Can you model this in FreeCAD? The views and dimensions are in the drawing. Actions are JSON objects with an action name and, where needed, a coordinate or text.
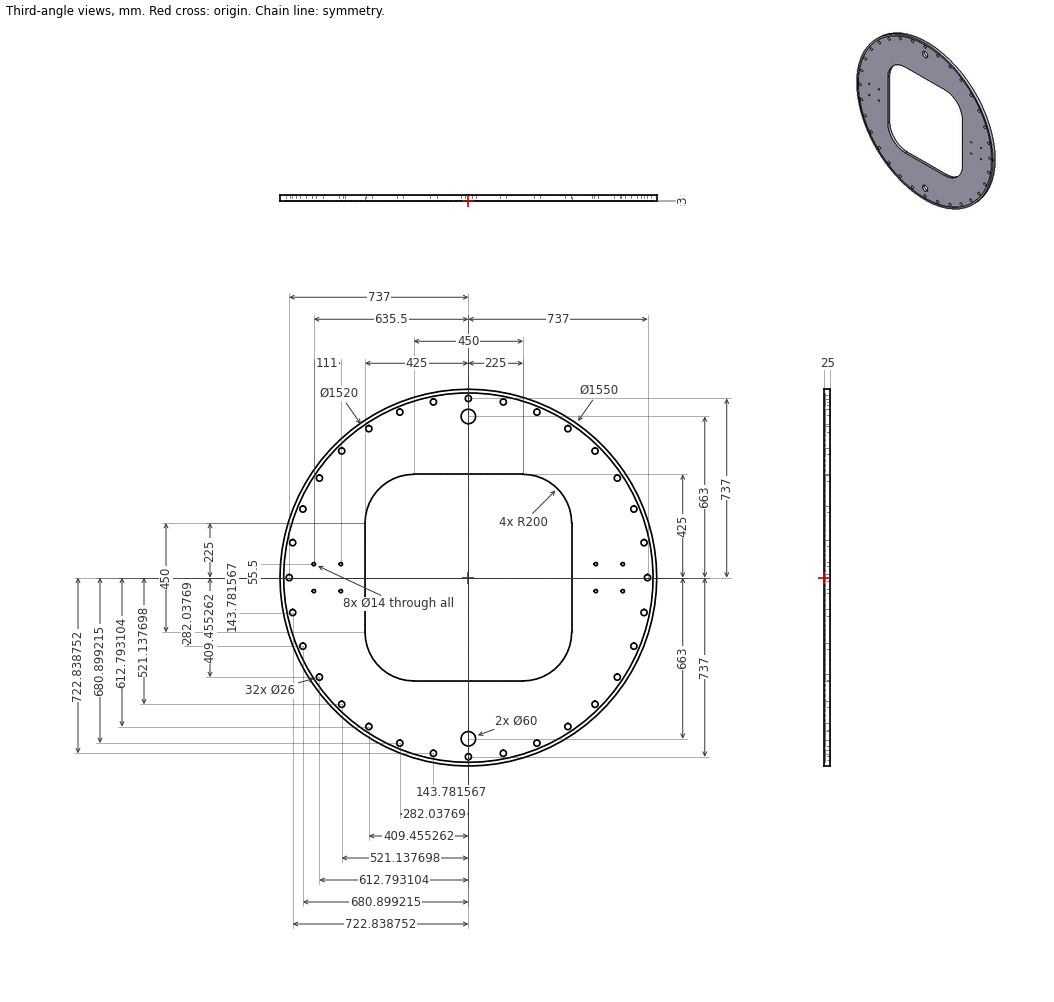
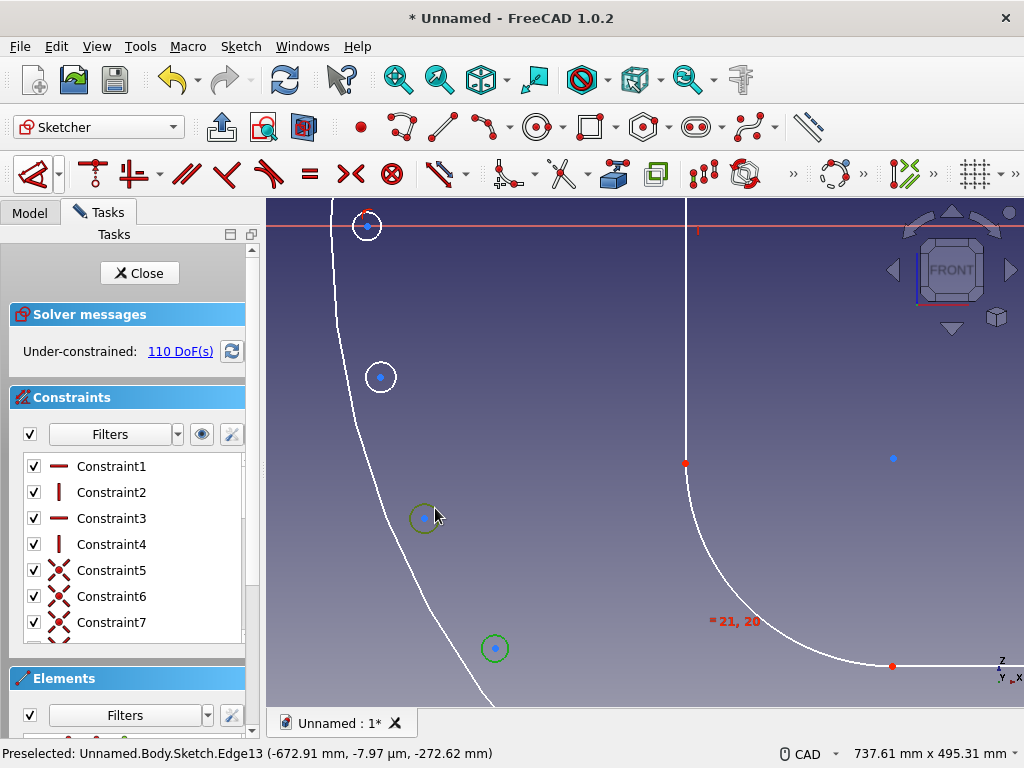
{"action": "left_click", "coordinate": [391, 367]}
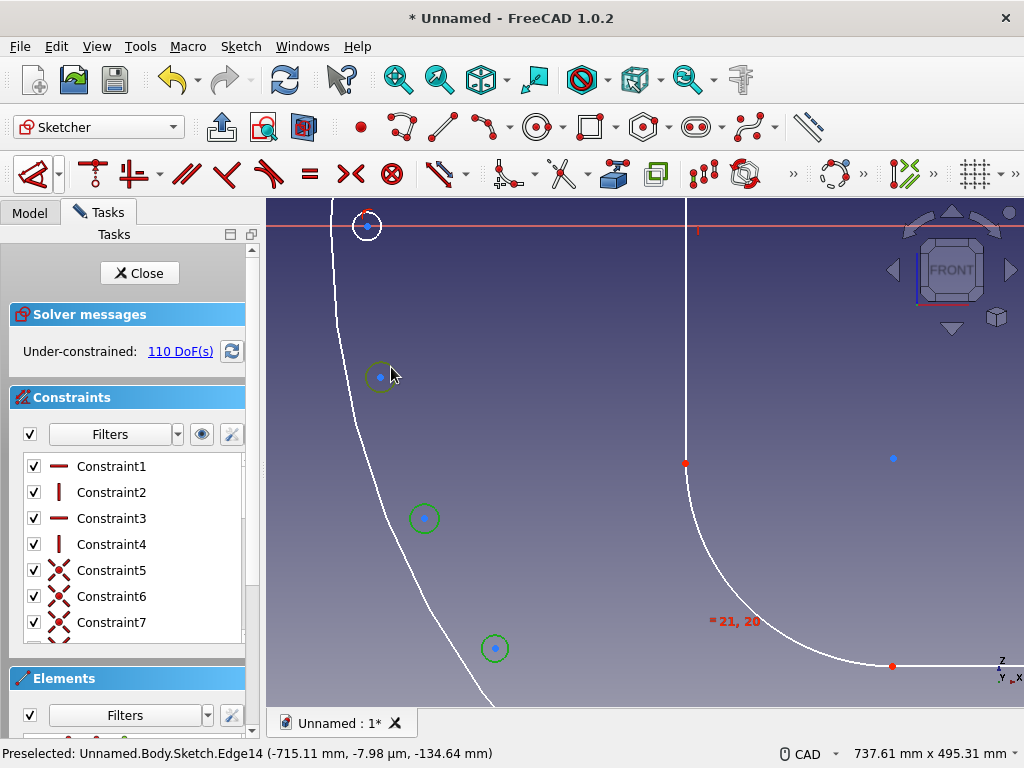
{"action": "scroll", "coordinate": [438, 510], "scroll_direction": "down", "scroll_amount": 8}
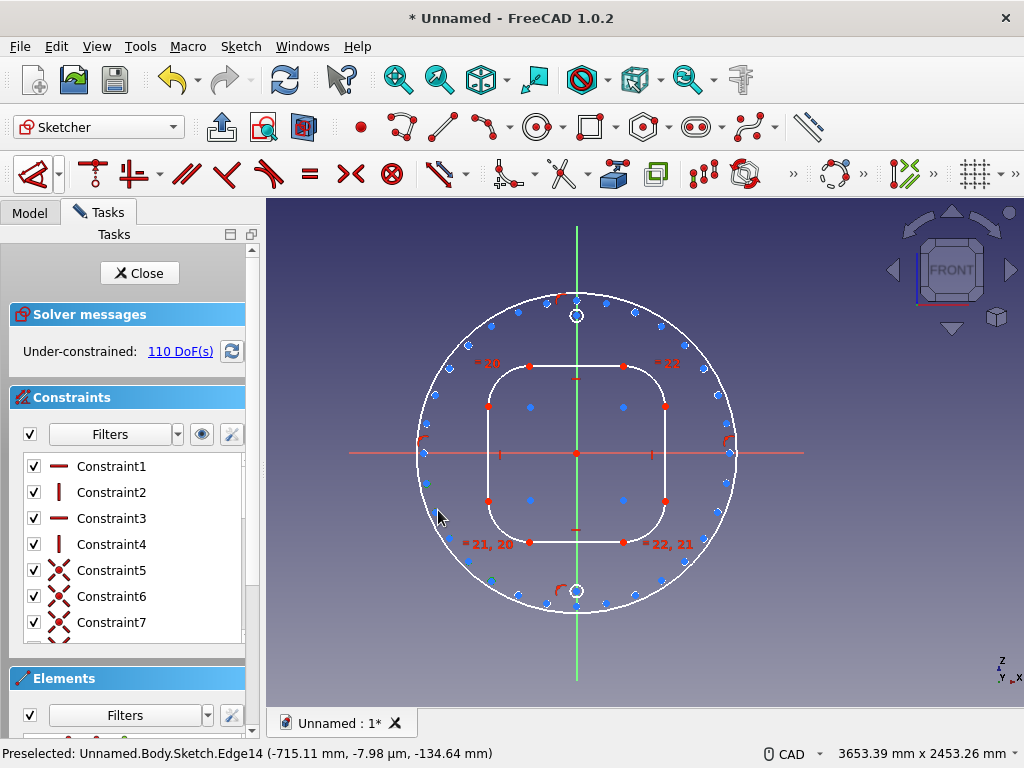
{"action": "scroll", "coordinate": [520, 593], "scroll_direction": "up", "scroll_amount": 8}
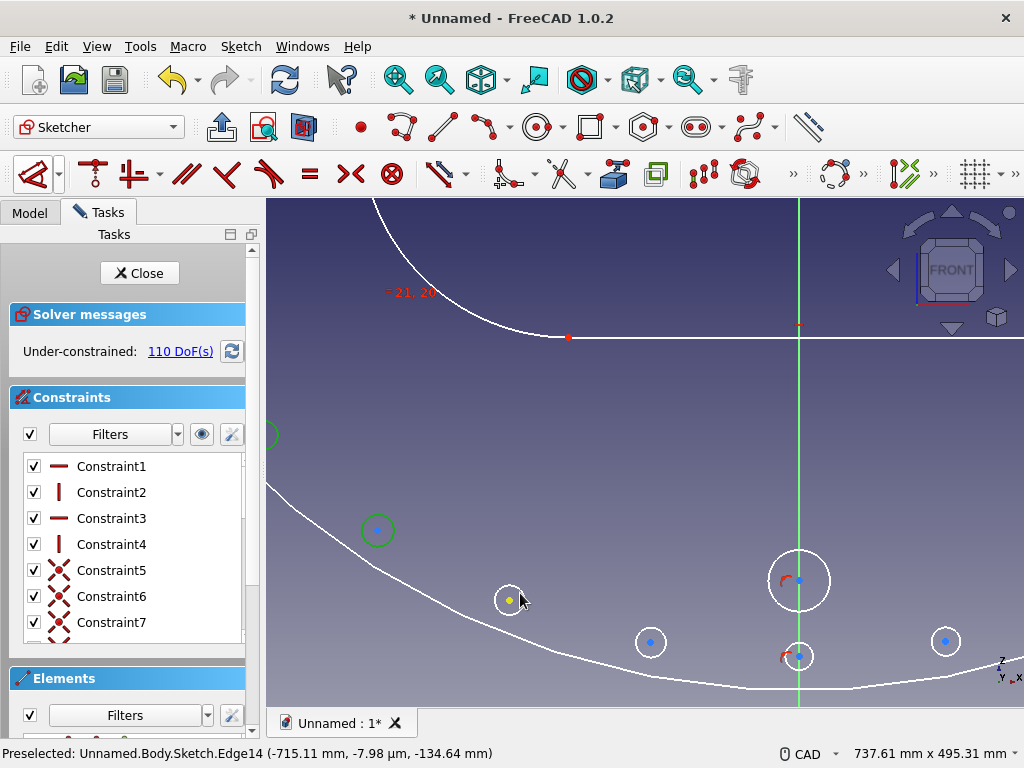
{"action": "left_click", "coordinate": [520, 590]}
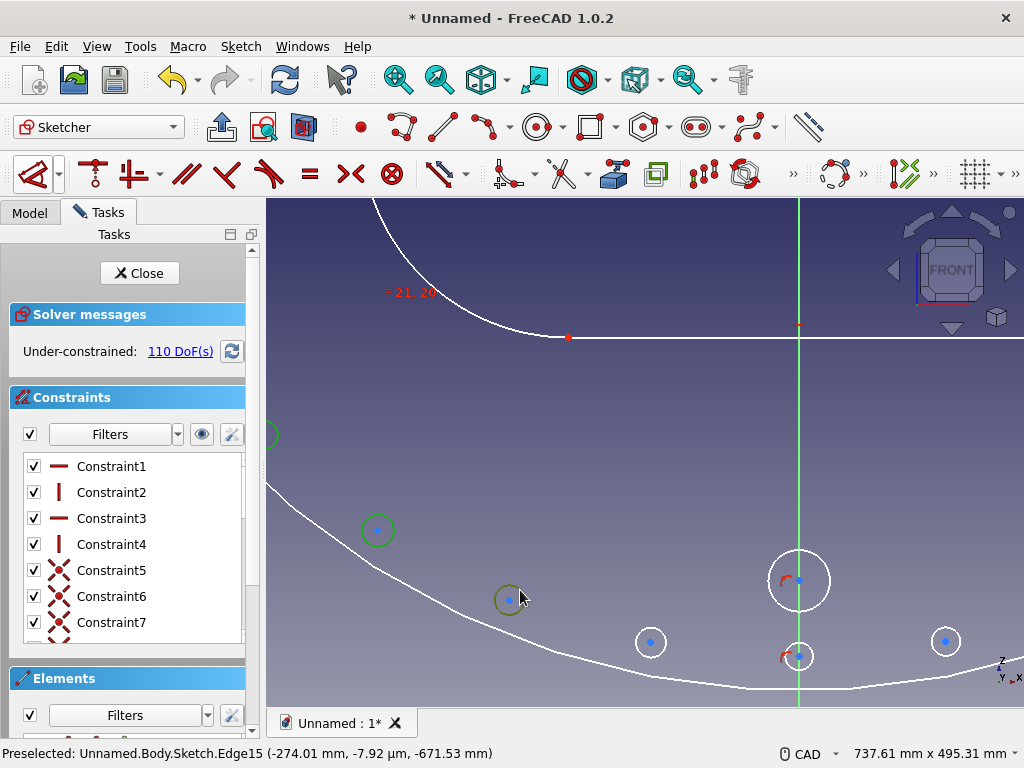
{"action": "left_click", "coordinate": [662, 632]}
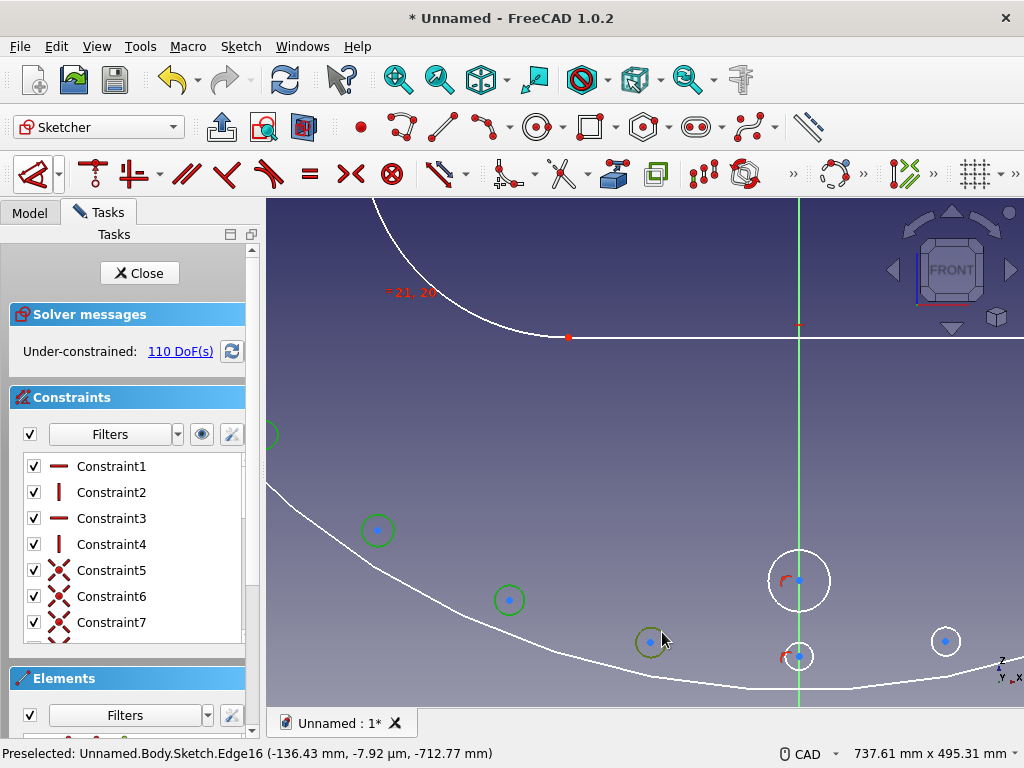
{"action": "scroll", "coordinate": [809, 647], "scroll_direction": "up", "scroll_amount": 2}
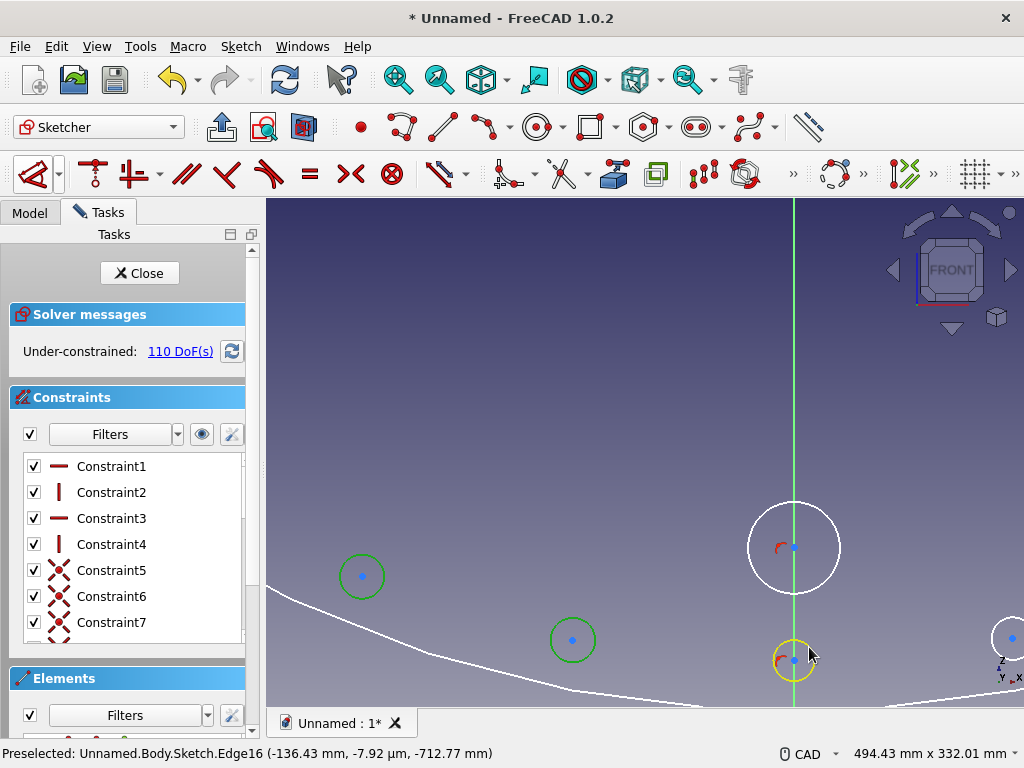
{"action": "left_click", "coordinate": [808, 646]}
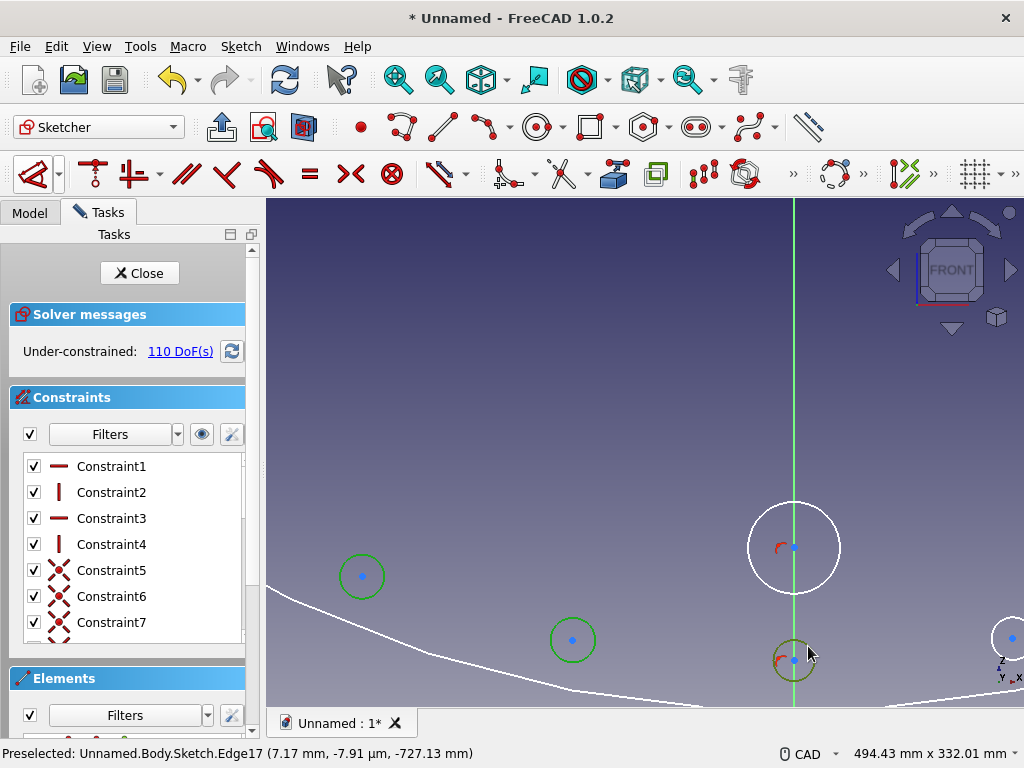
{"action": "scroll", "coordinate": [542, 597], "scroll_direction": "down", "scroll_amount": 10}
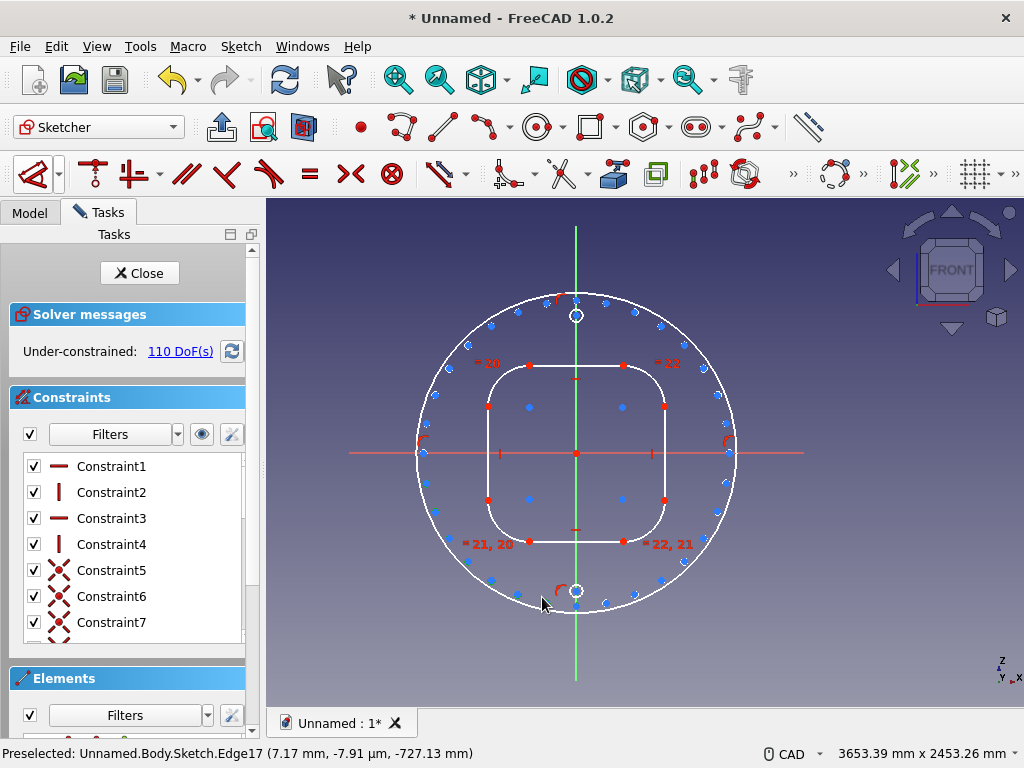
{"action": "scroll", "coordinate": [426, 451], "scroll_direction": "up", "scroll_amount": 10}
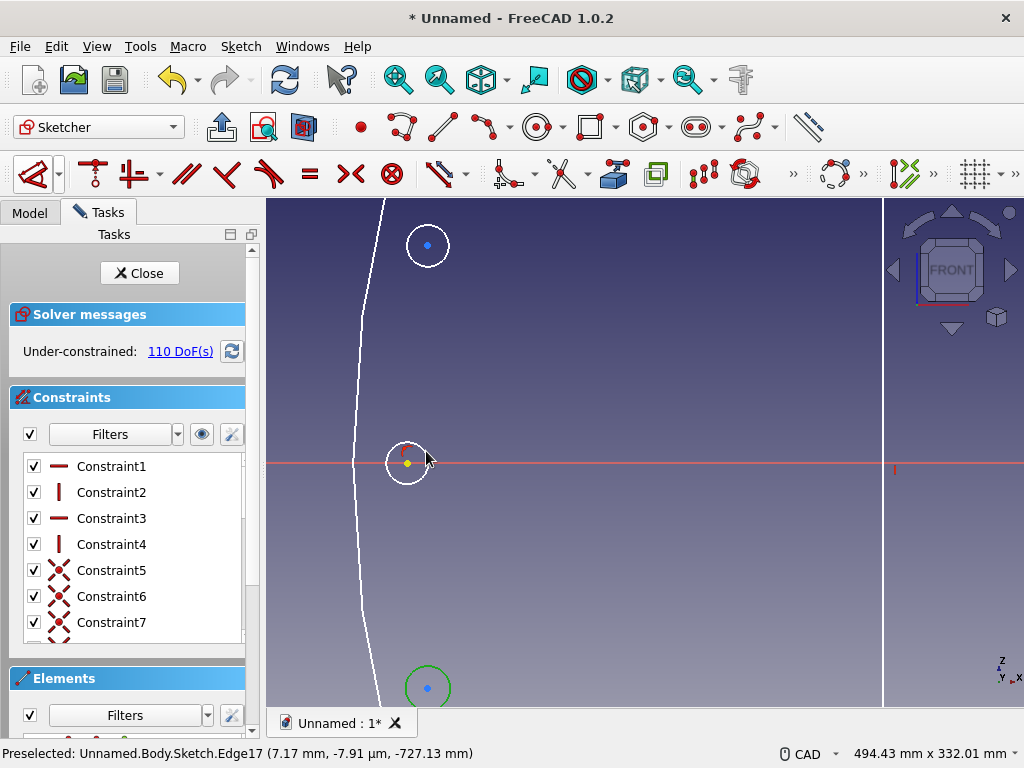
{"action": "left_click", "coordinate": [422, 448]}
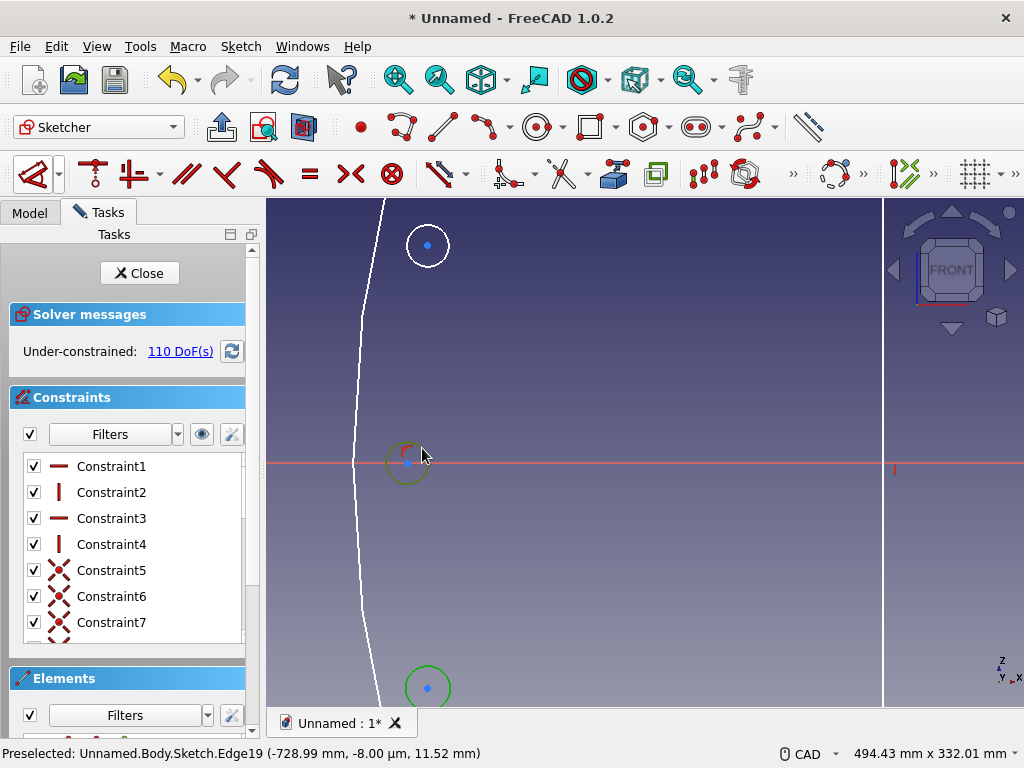
{"action": "left_click", "coordinate": [443, 231]}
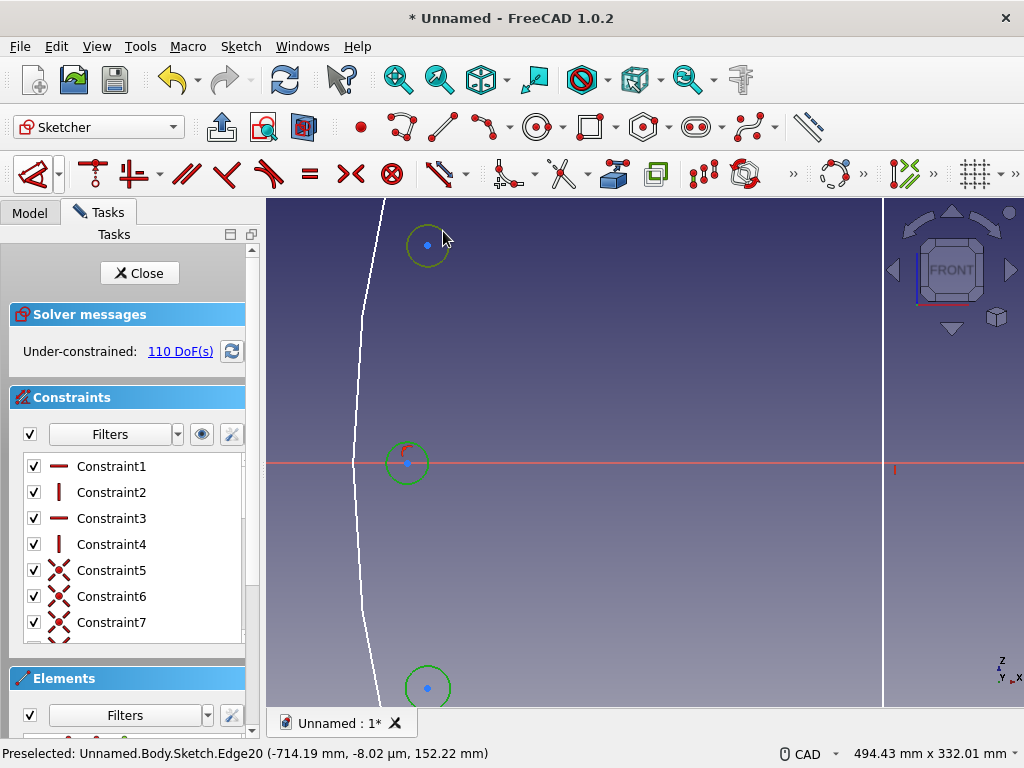
{"action": "scroll", "coordinate": [426, 451], "scroll_direction": "down", "scroll_amount": 10}